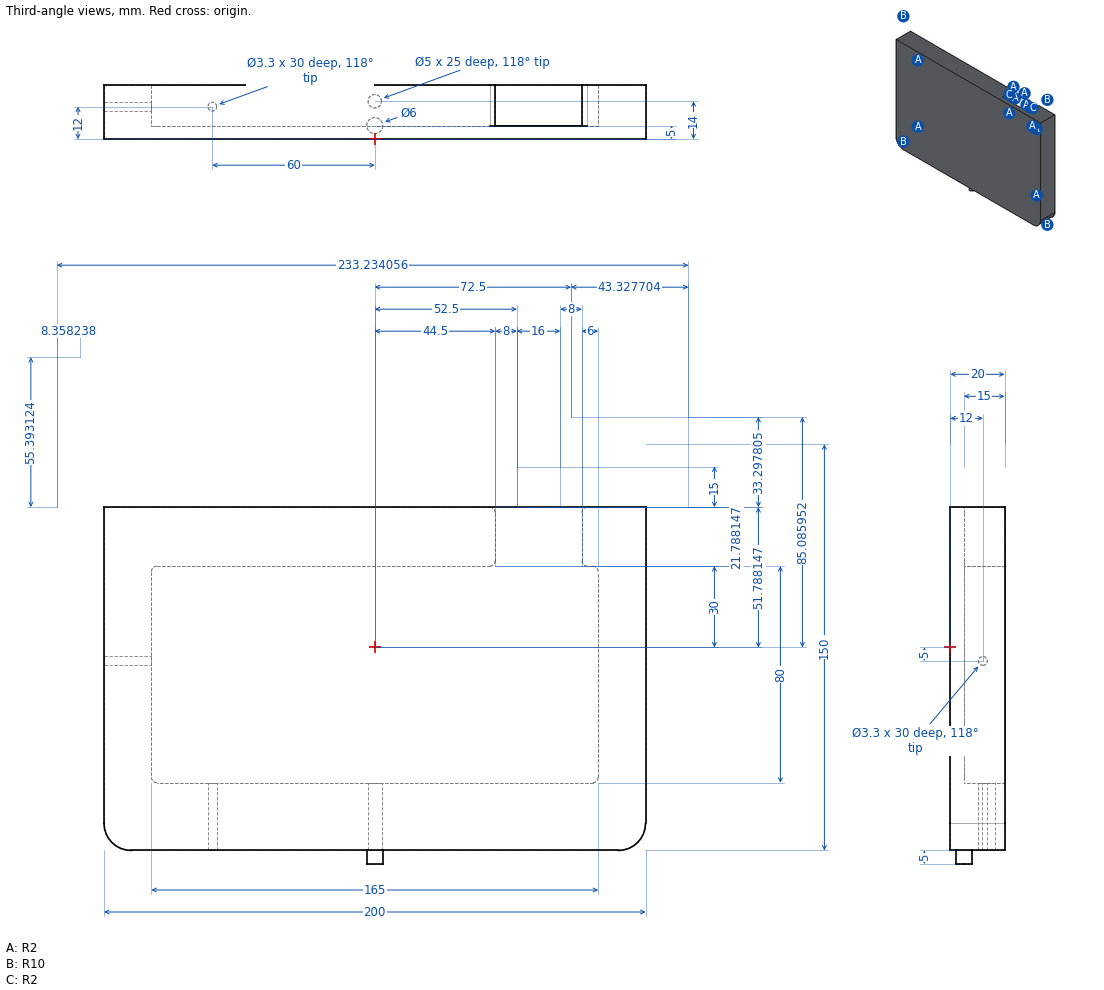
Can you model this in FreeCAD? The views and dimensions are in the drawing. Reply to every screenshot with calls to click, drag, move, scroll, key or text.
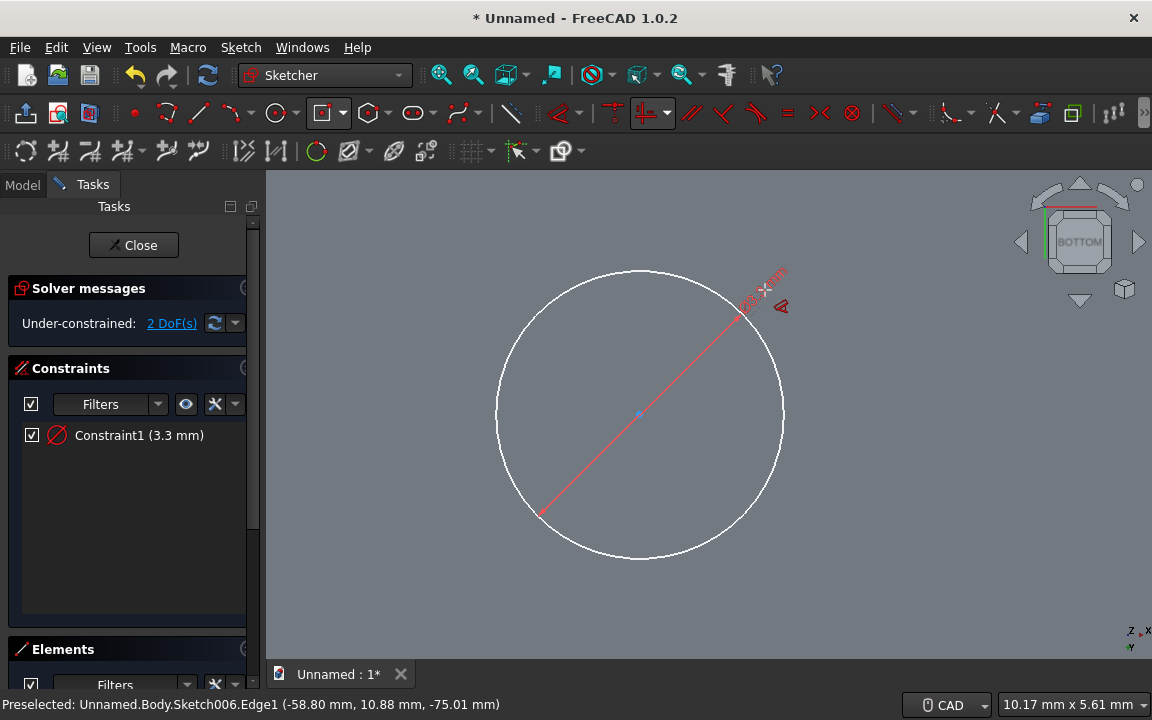
click(640, 415)
click(813, 449)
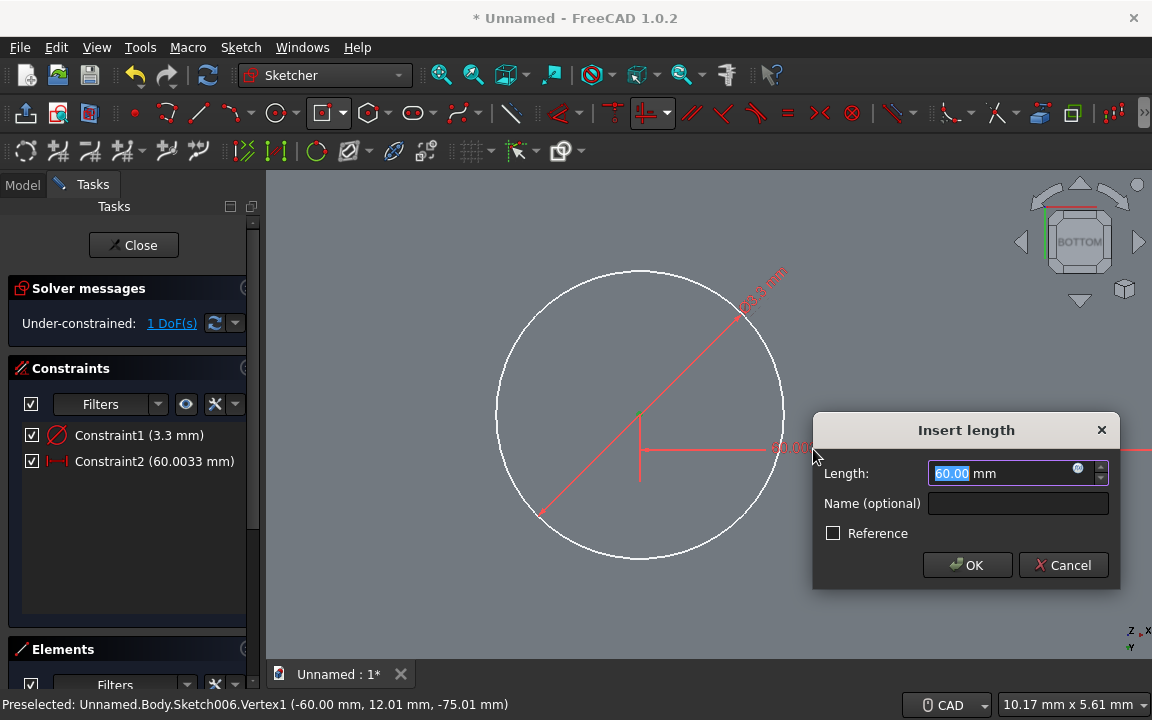
text(60)
key(Return)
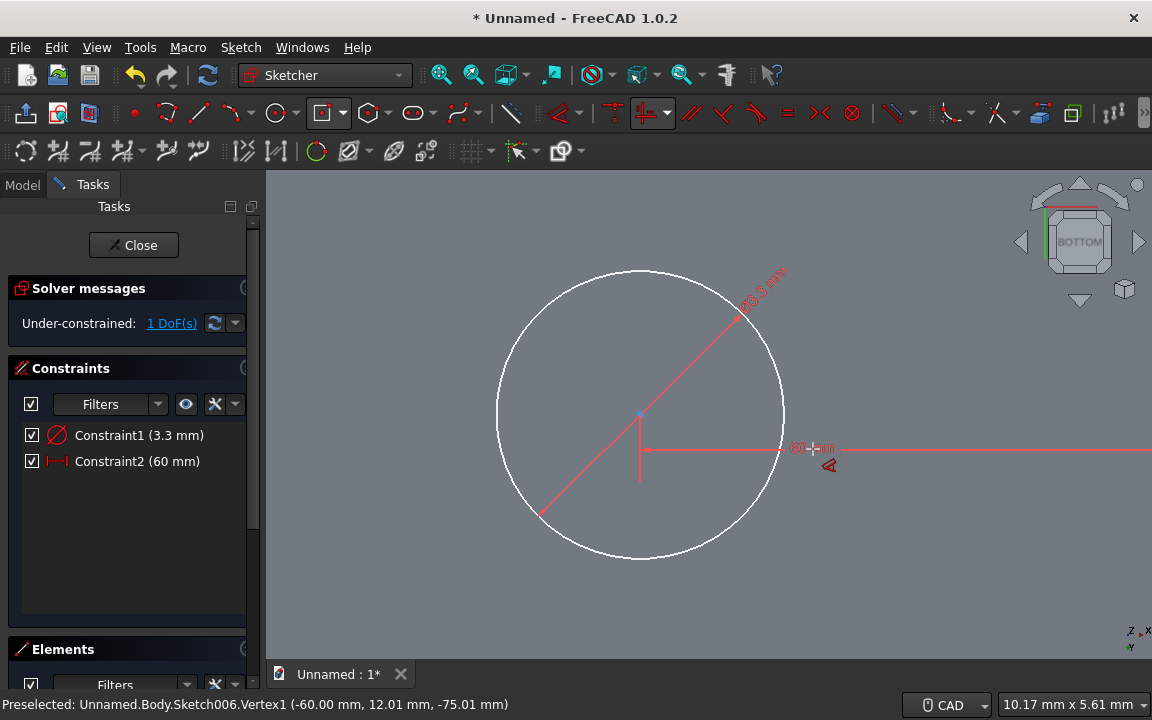
click(640, 415)
click(606, 306)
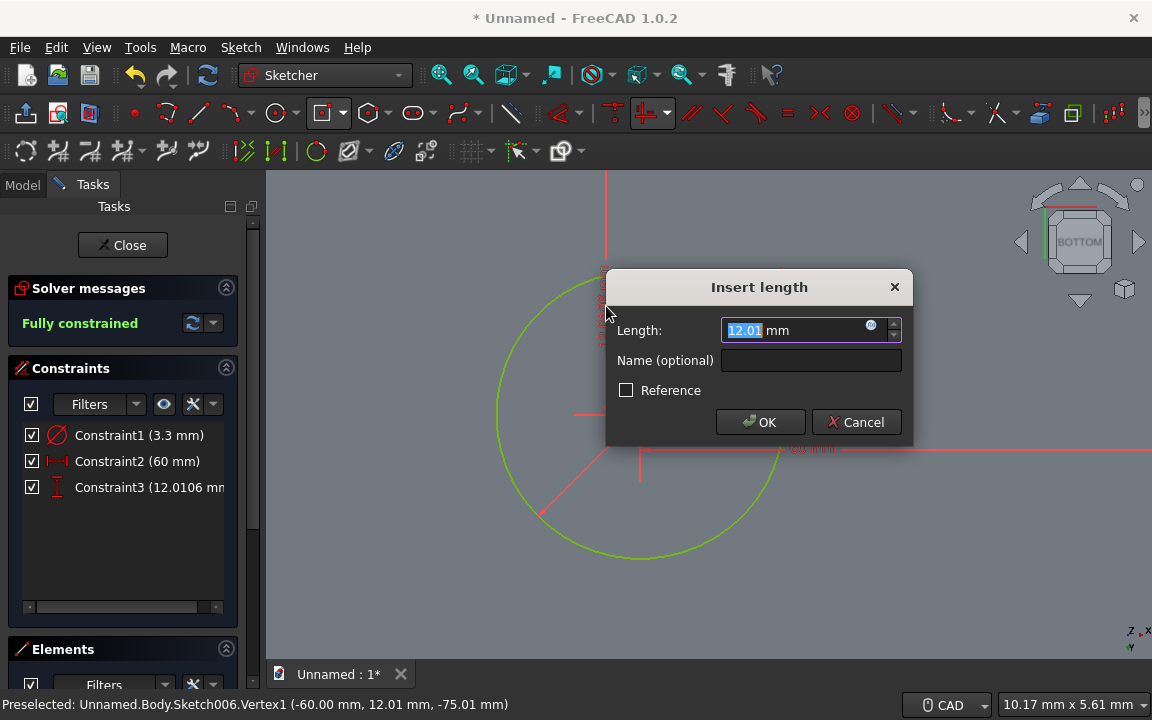
text(12)
key(Return)
key(Escape)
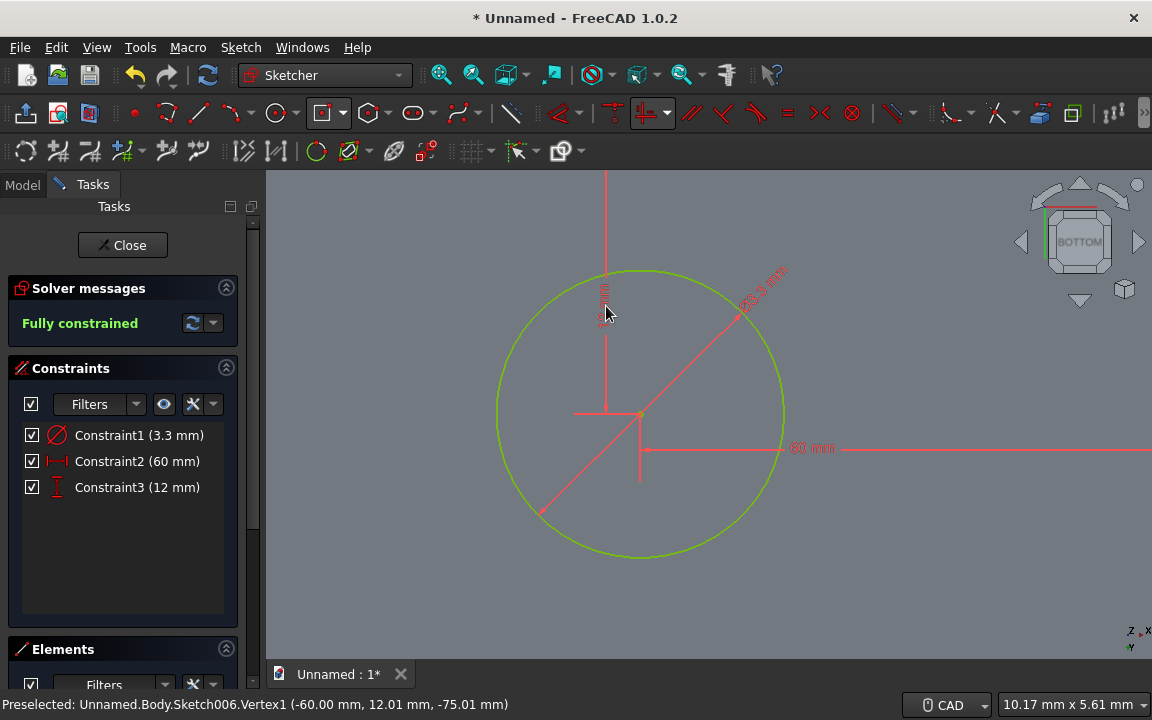
click(123, 245)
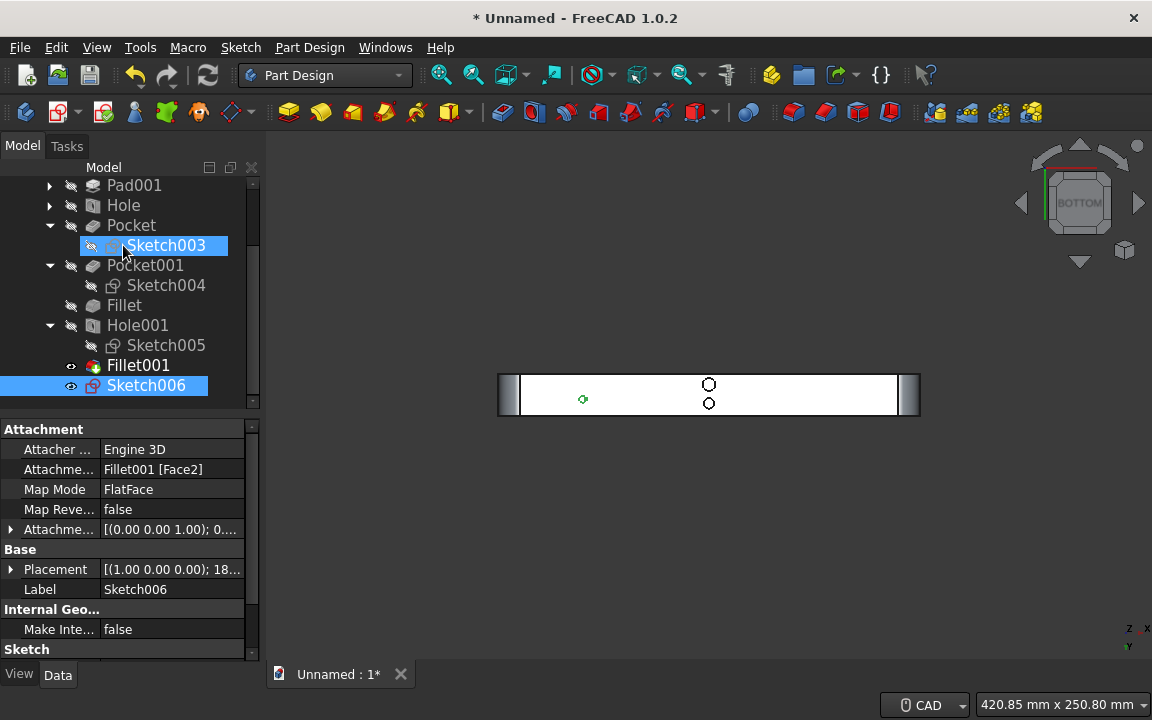
click(536, 112)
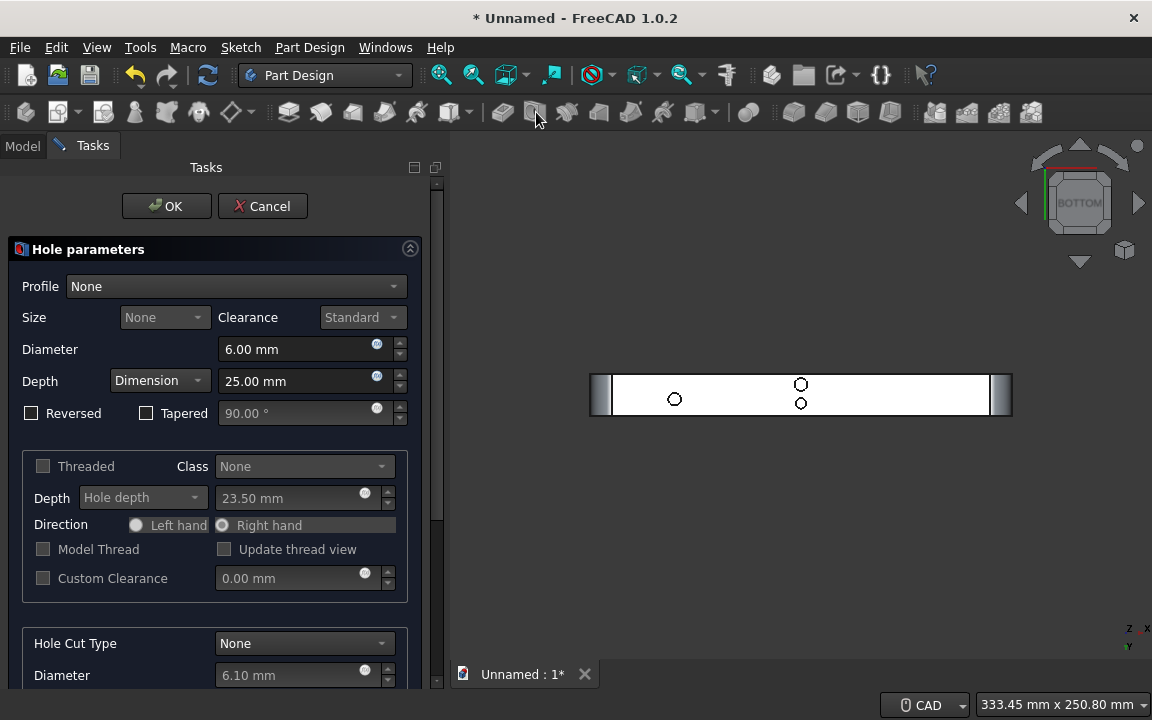
triple_click(305, 349)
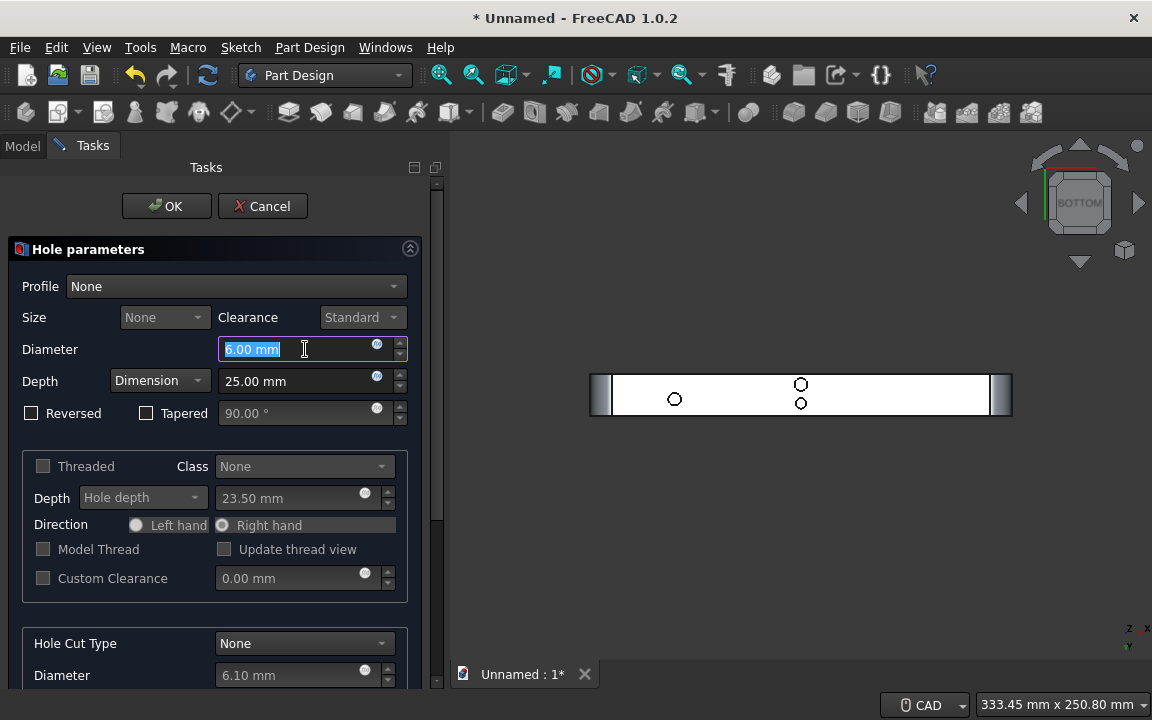
text(3.3)
key(Tab)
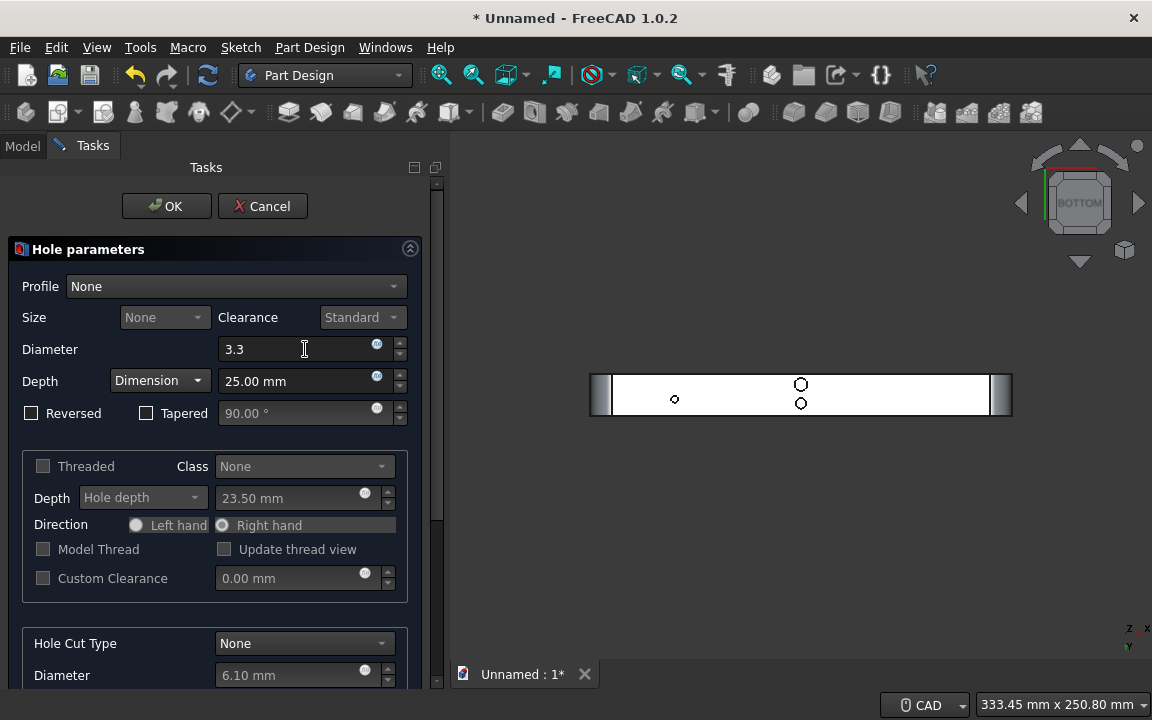
triple_click(305, 381)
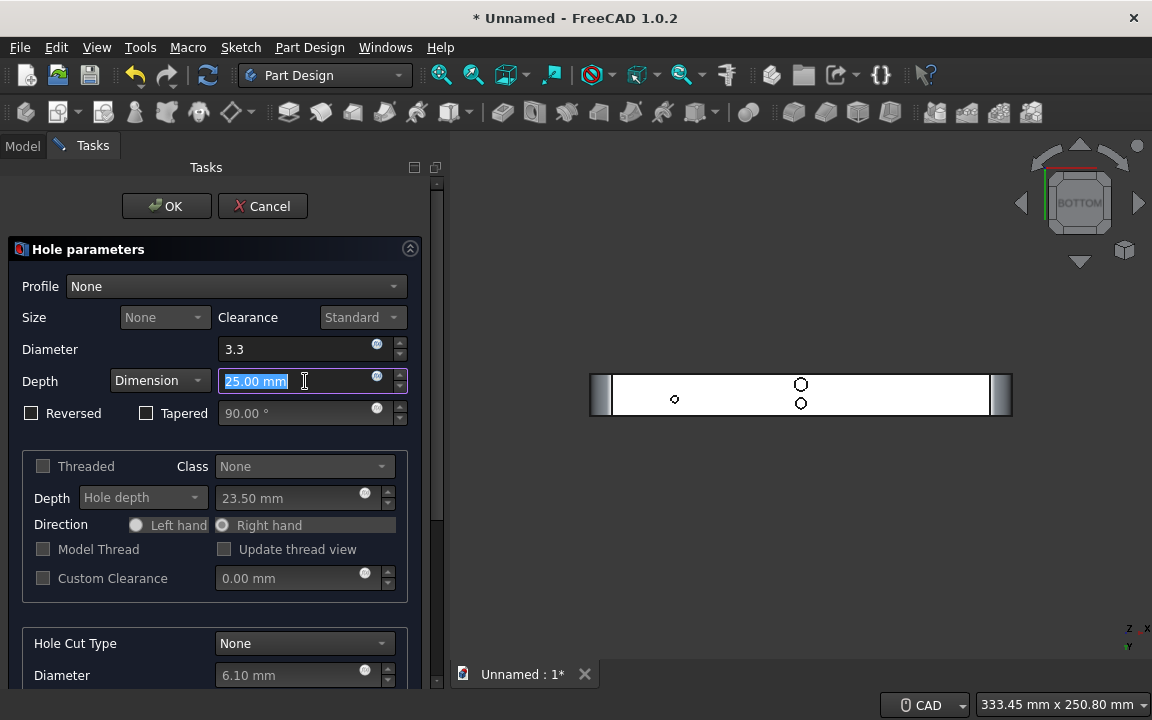
text(30)
key(Tab)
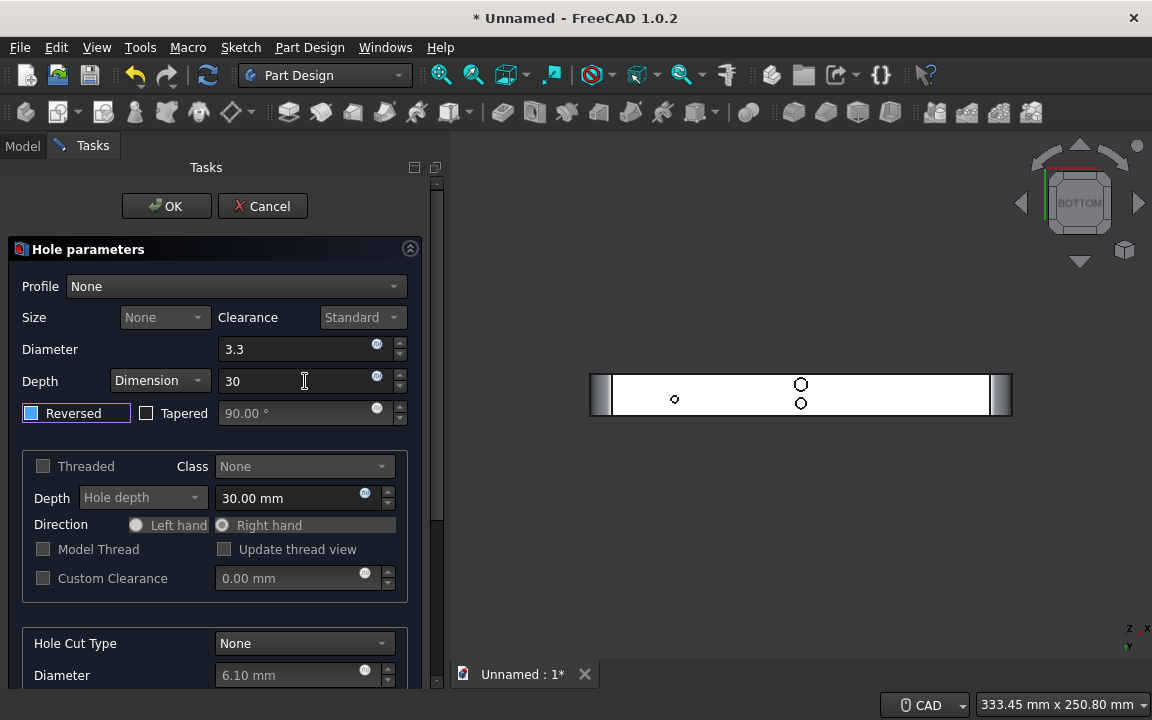
click(167, 206)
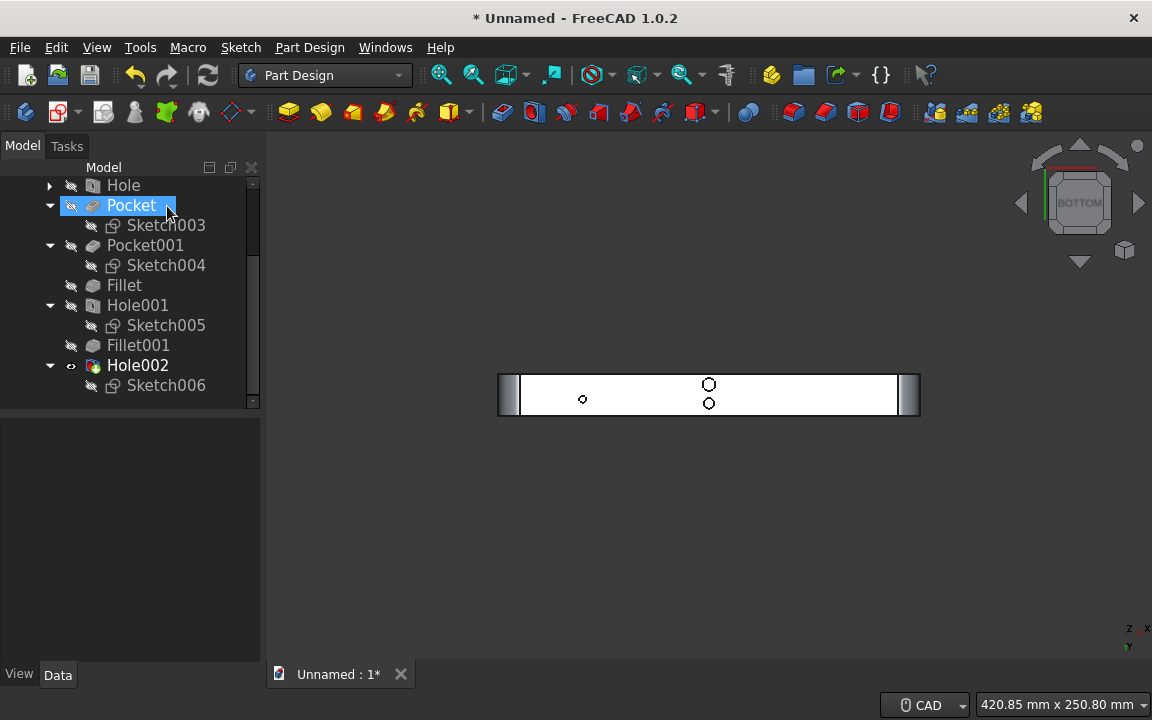
key(4)